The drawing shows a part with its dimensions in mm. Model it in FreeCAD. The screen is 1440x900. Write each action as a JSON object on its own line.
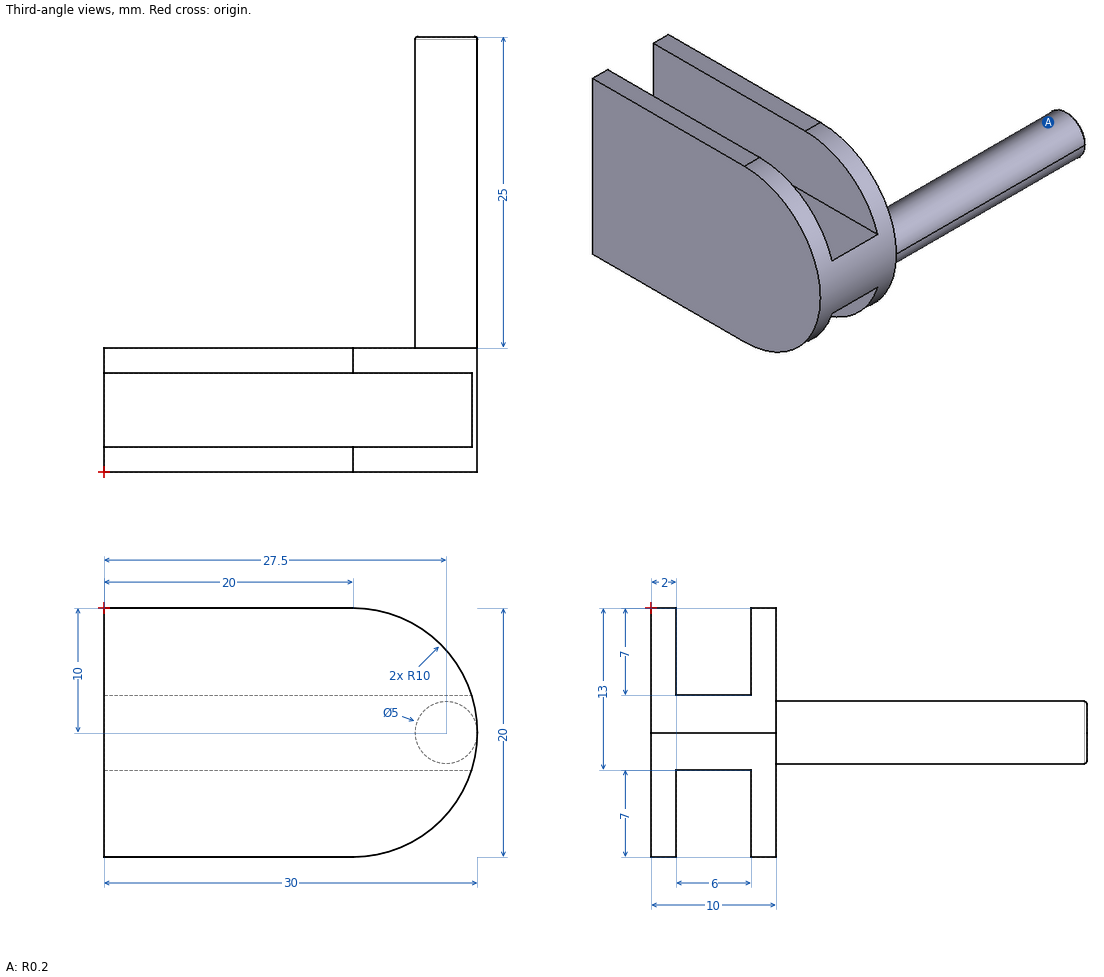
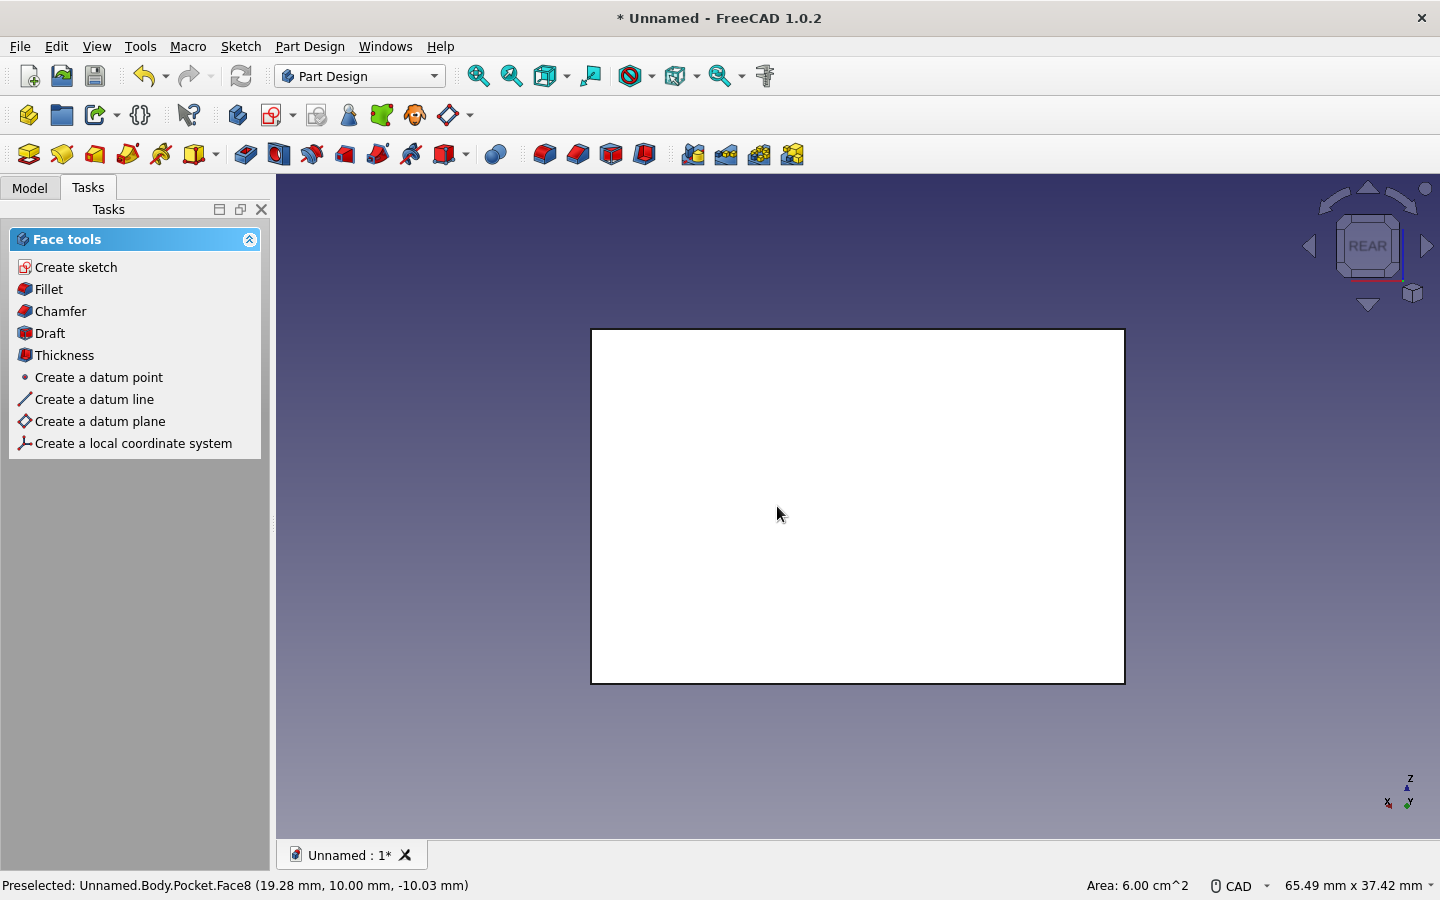
{"action": "left_click", "coordinate": [270, 116]}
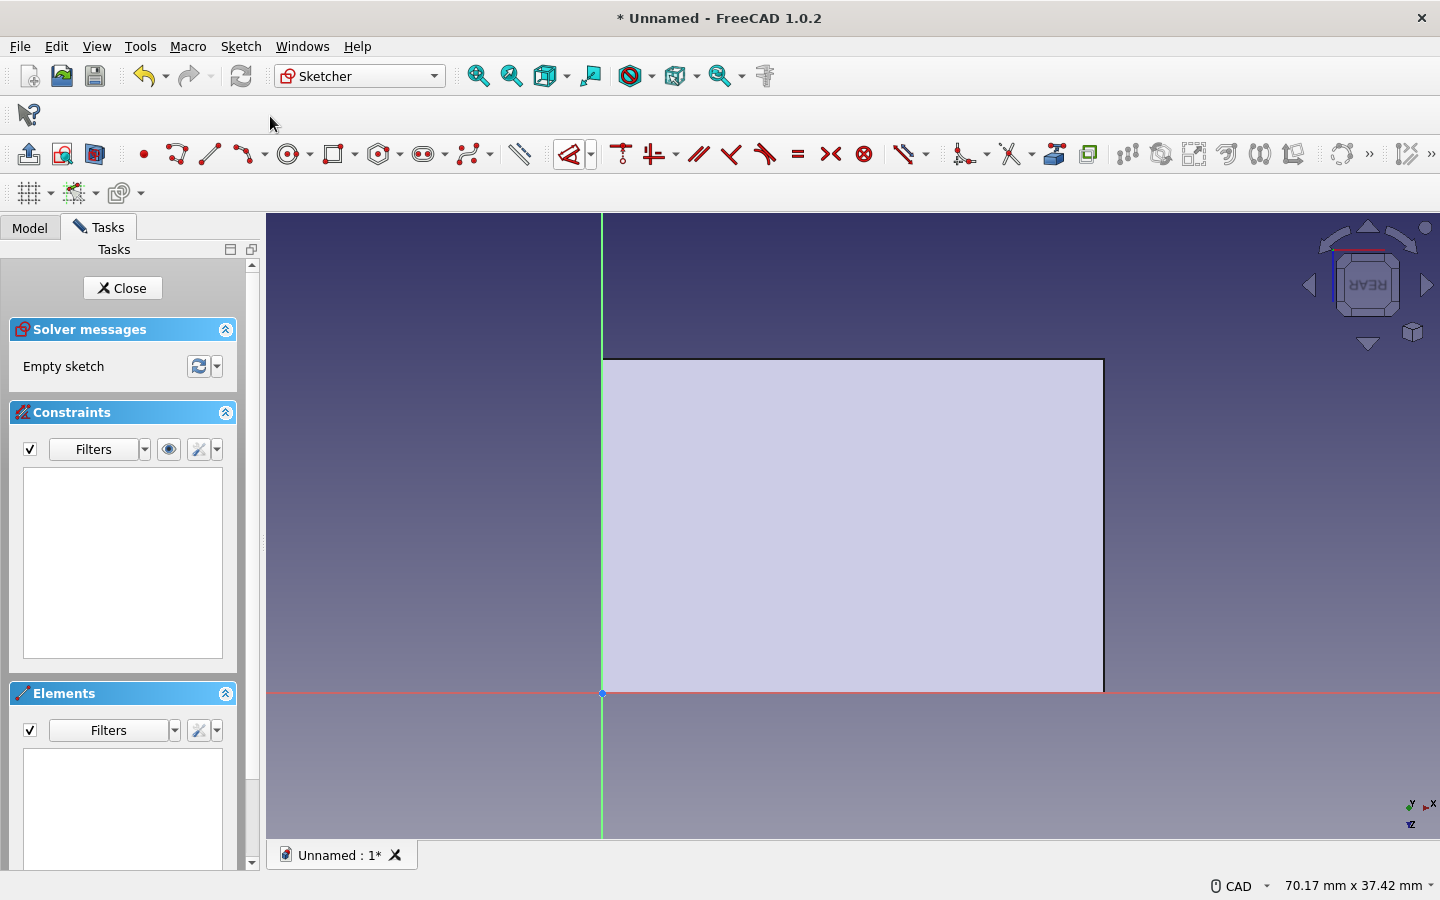
{"action": "left_click", "coordinate": [177, 154]}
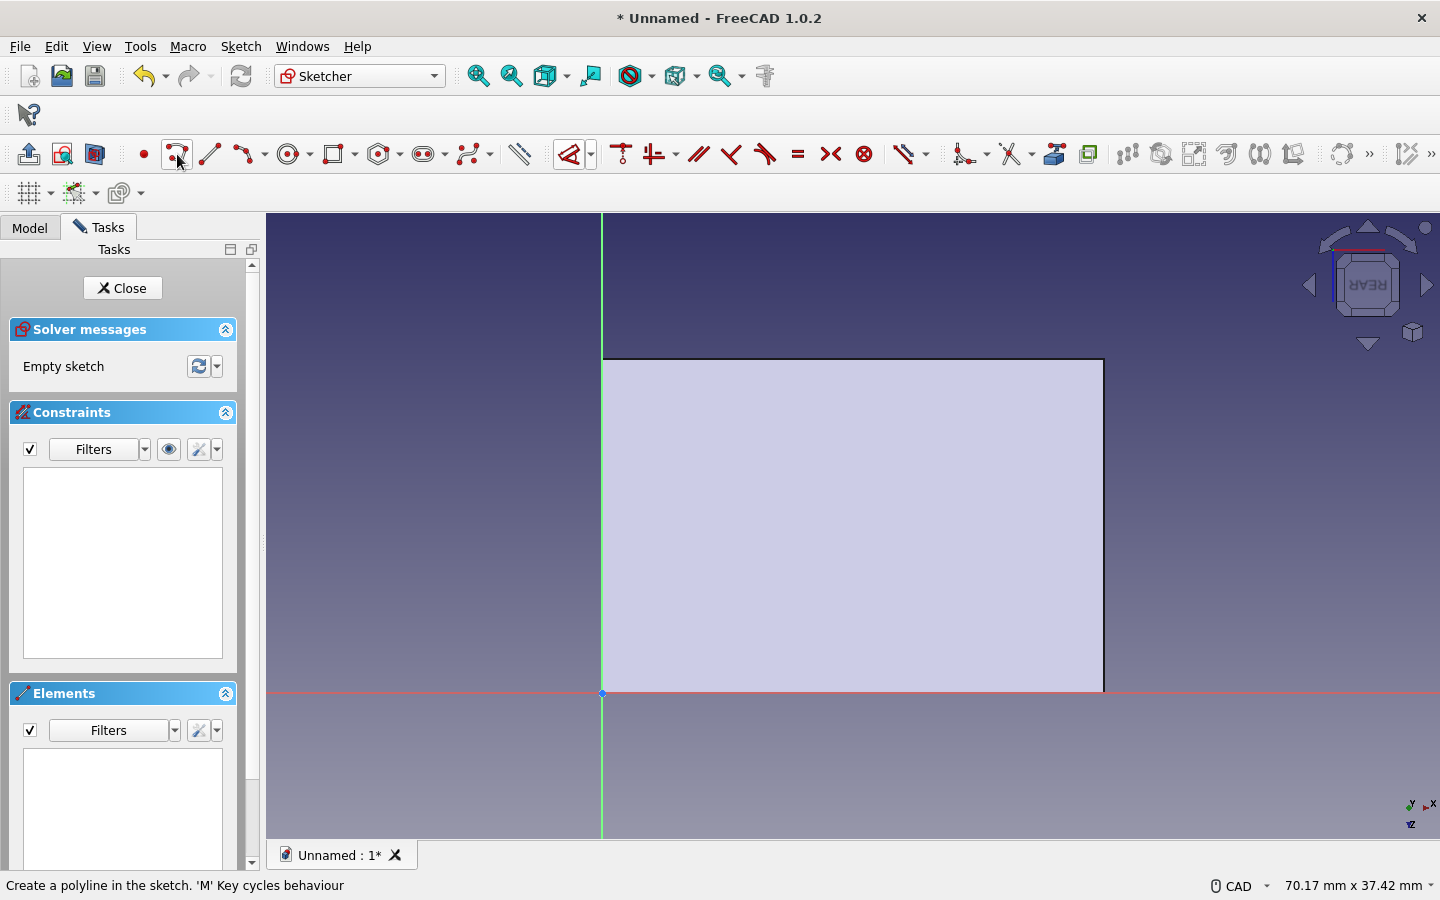
{"action": "left_click", "coordinate": [937, 693]}
{"action": "left_click", "coordinate": [1104, 684]}
{"action": "left_click", "coordinate": [1104, 526]}
{"action": "right_click", "coordinate": [1104, 526]}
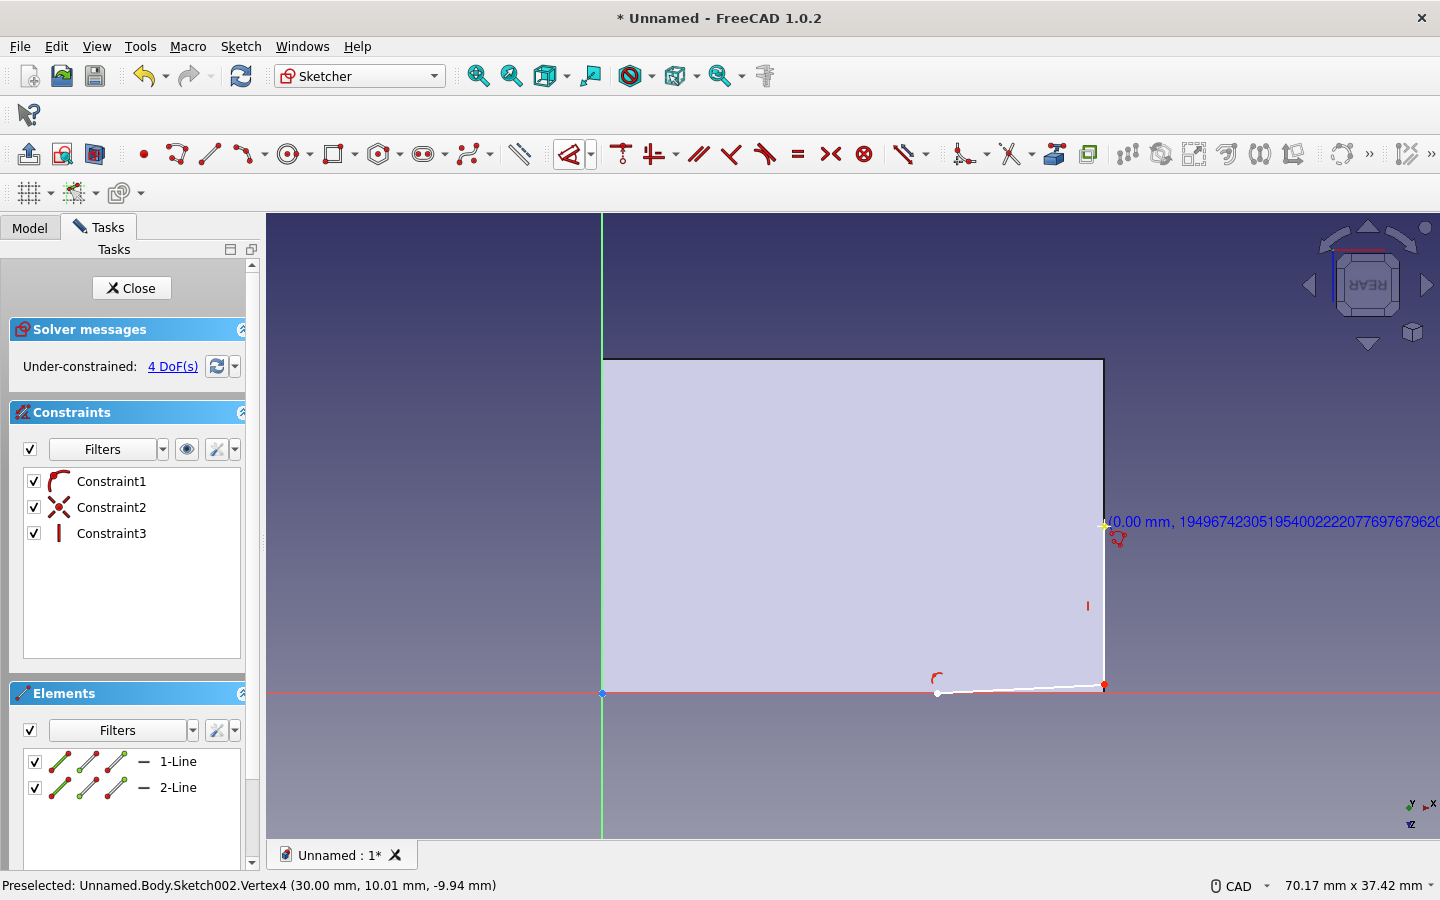
{"action": "left_click", "coordinate": [242, 154]}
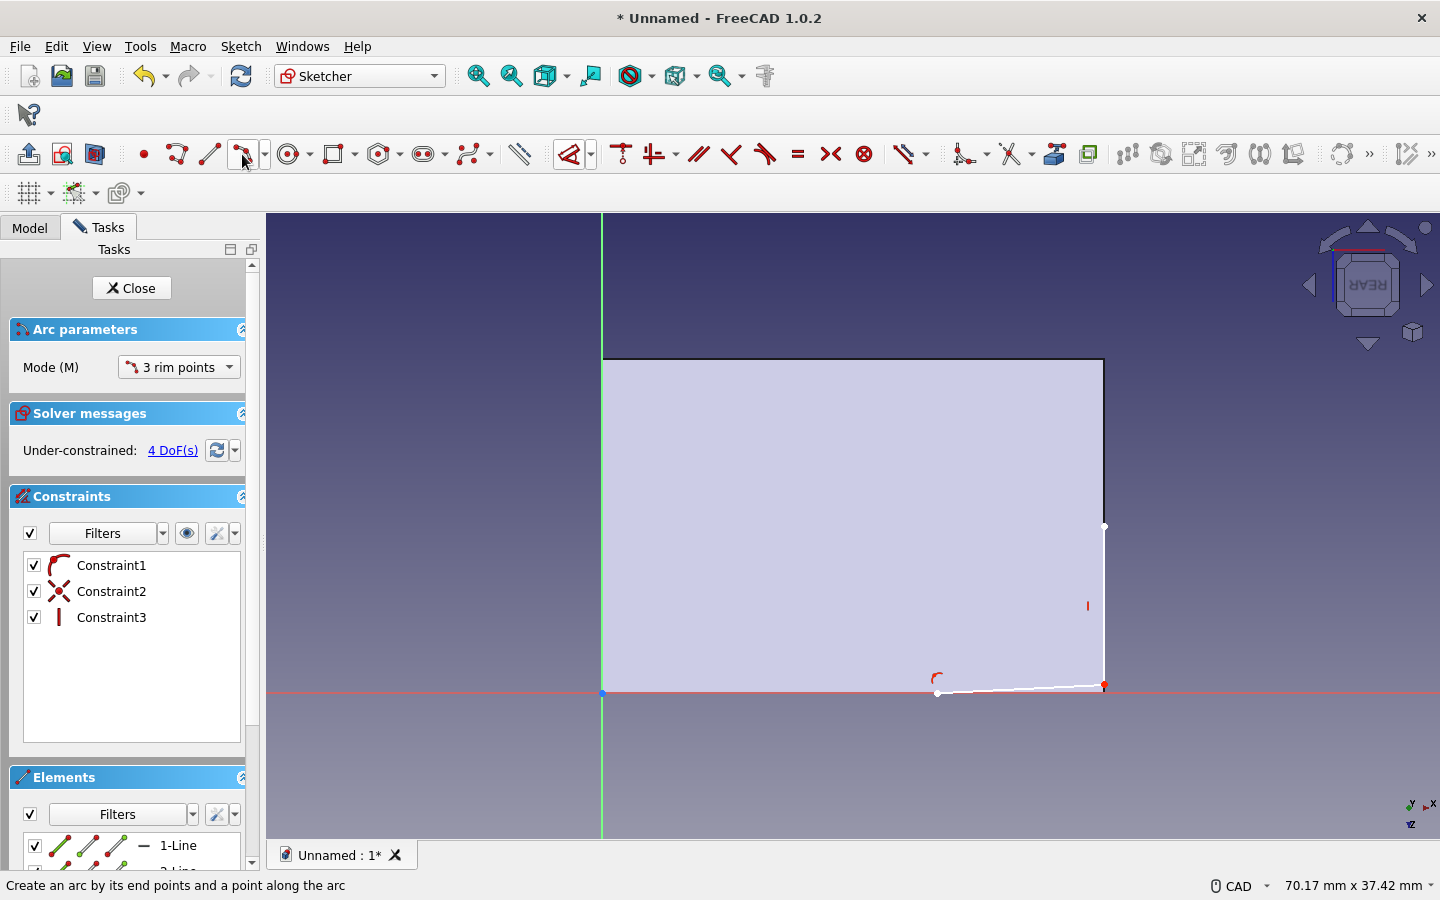
{"action": "left_click", "coordinate": [1104, 527]}
{"action": "left_click", "coordinate": [937, 693]}
{"action": "left_click", "coordinate": [1055, 644]}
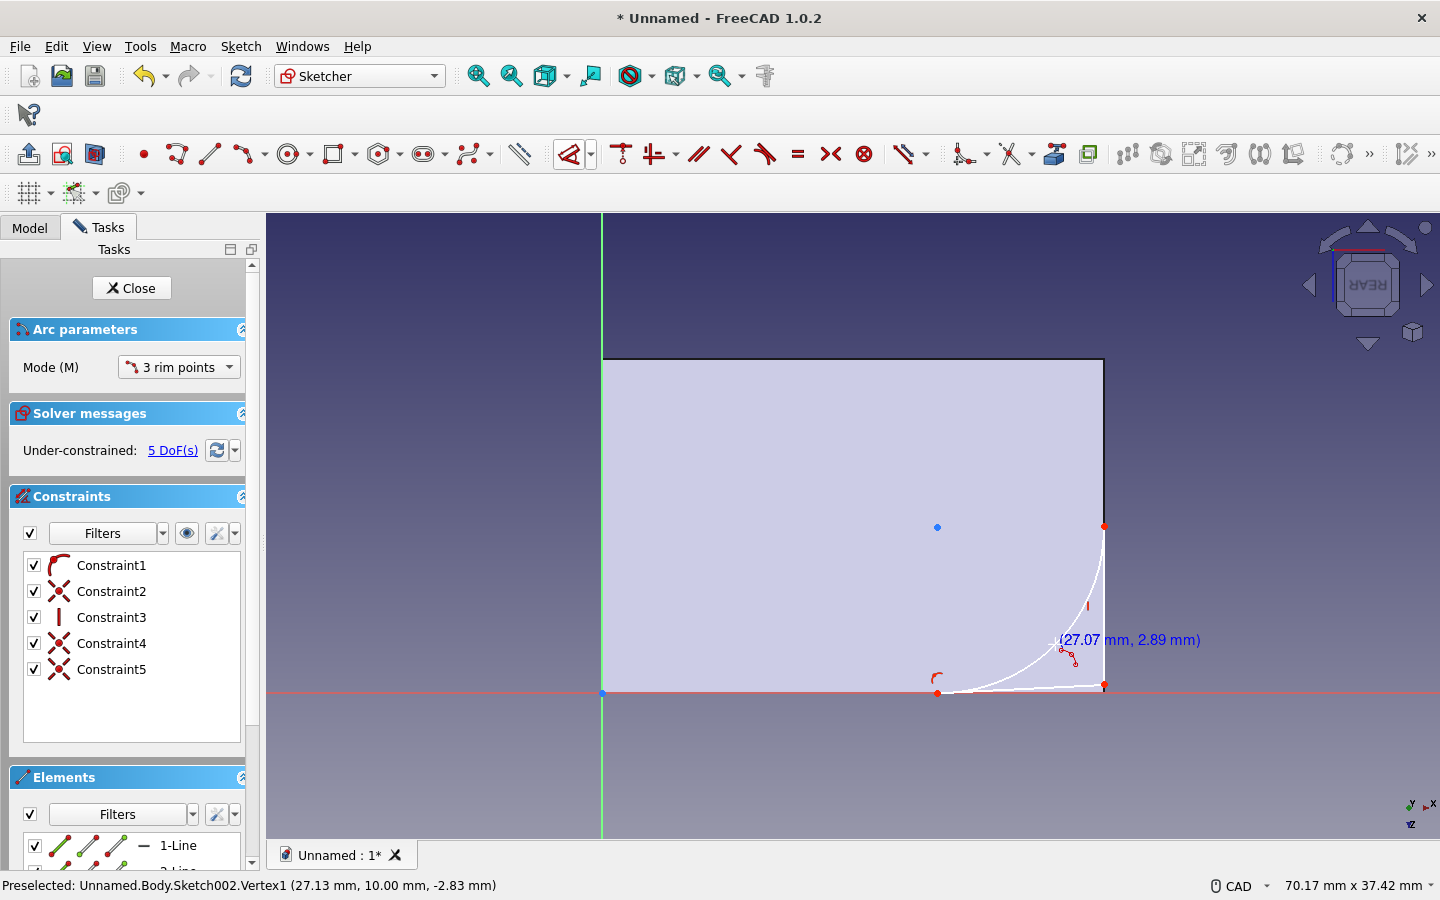
{"action": "left_click", "coordinate": [177, 154]}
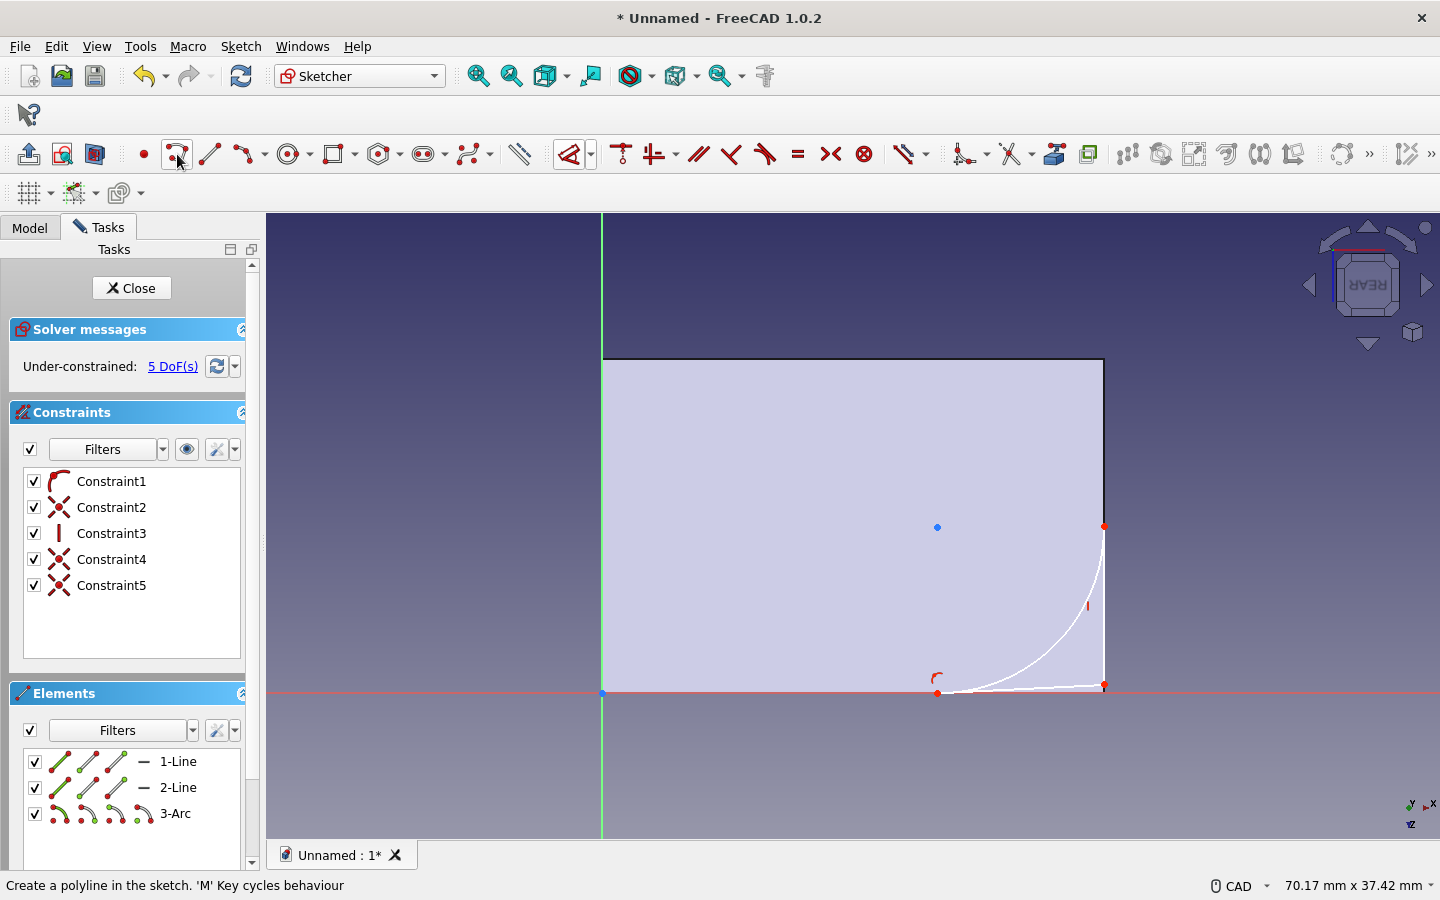
{"action": "left_click", "coordinate": [1104, 527]}
{"action": "left_click", "coordinate": [1104, 359]}
{"action": "left_click", "coordinate": [937, 359]}
{"action": "right_click", "coordinate": [937, 359]}